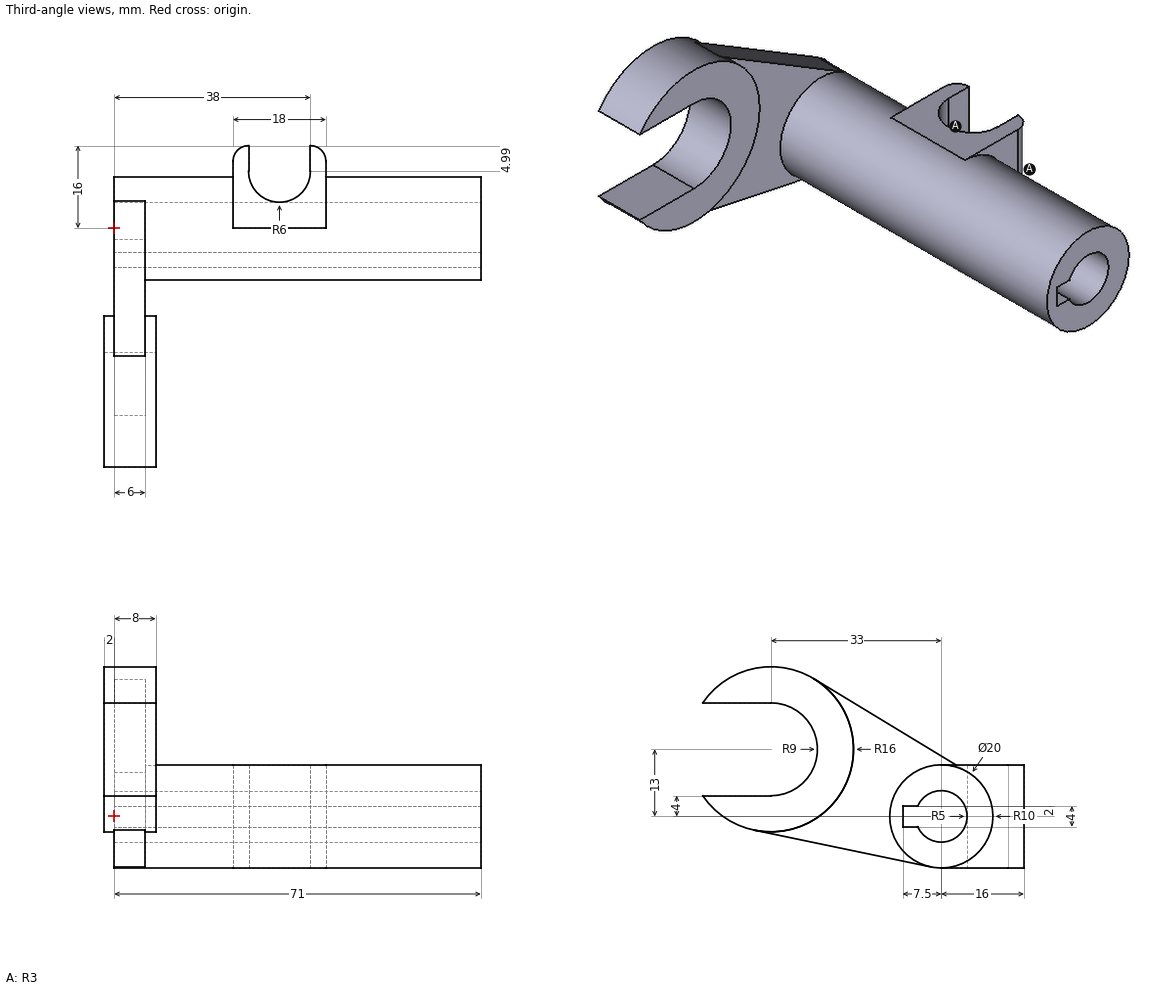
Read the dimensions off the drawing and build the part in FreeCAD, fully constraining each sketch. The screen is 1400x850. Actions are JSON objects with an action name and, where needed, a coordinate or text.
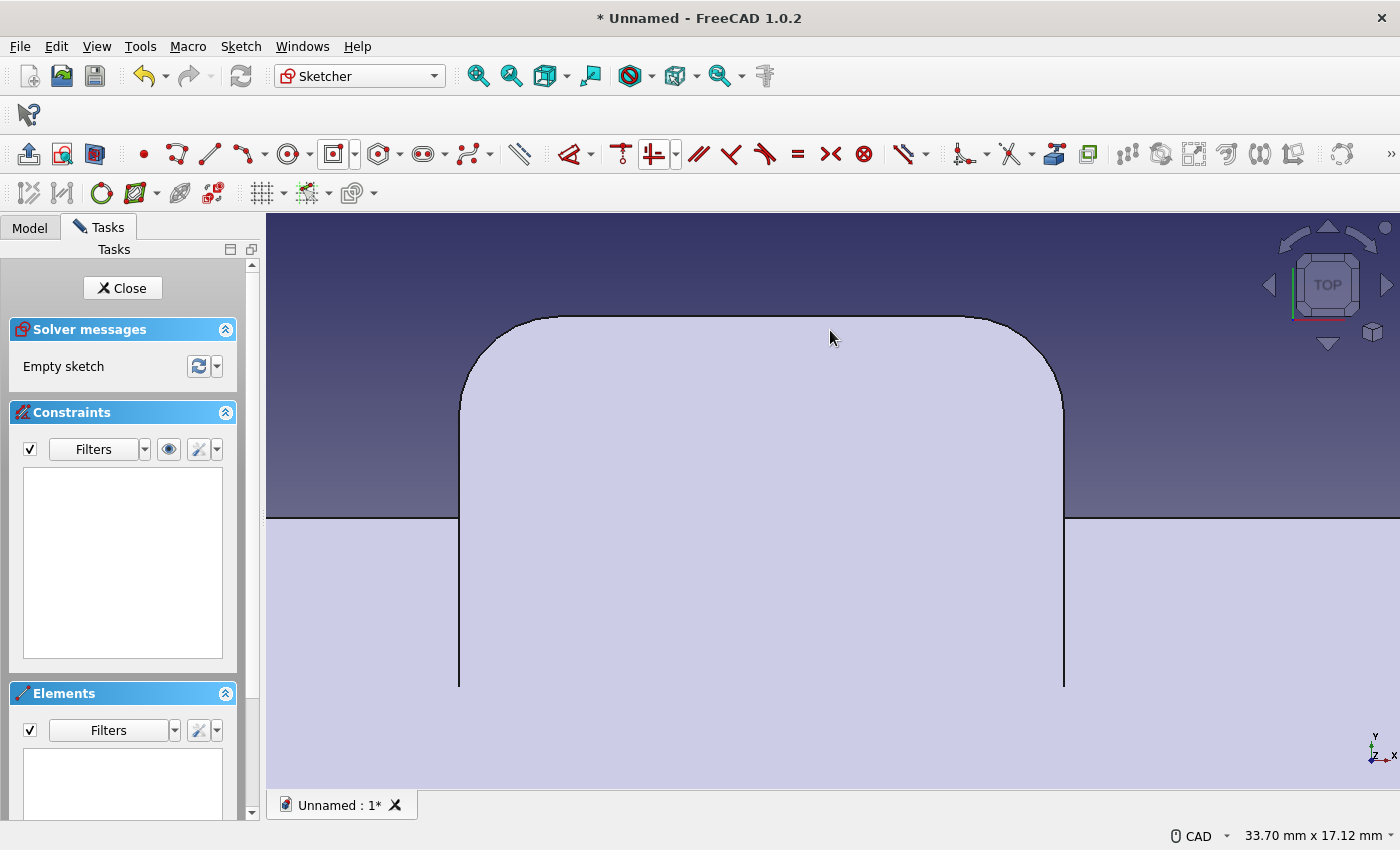
{"action": "left_click", "coordinate": [177, 154]}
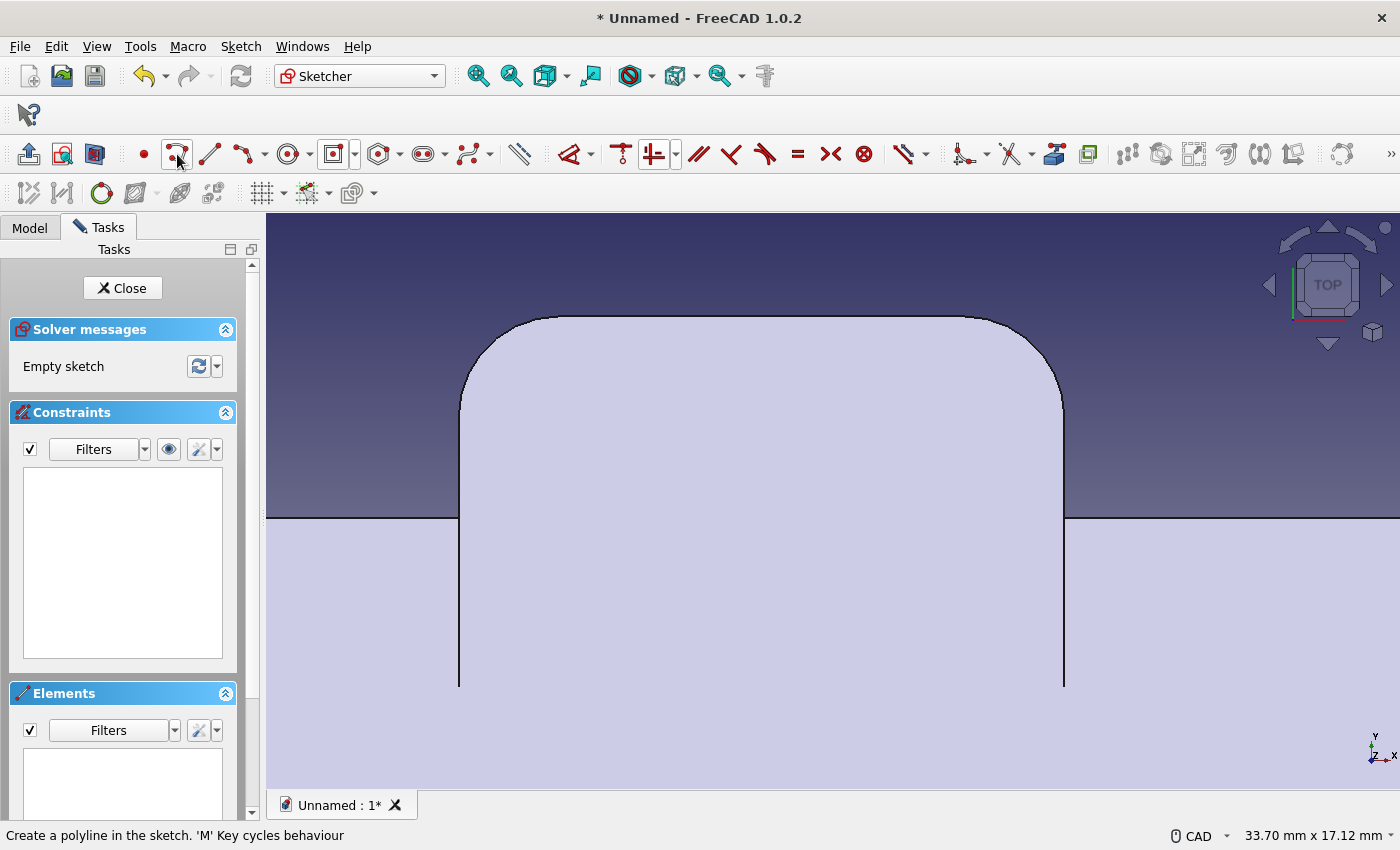
{"action": "left_click", "coordinate": [963, 484]}
{"action": "left_click", "coordinate": [963, 316]}
{"action": "left_click", "coordinate": [560, 316]}
{"action": "left_click", "coordinate": [560, 484]}
{"action": "right_click", "coordinate": [560, 484]}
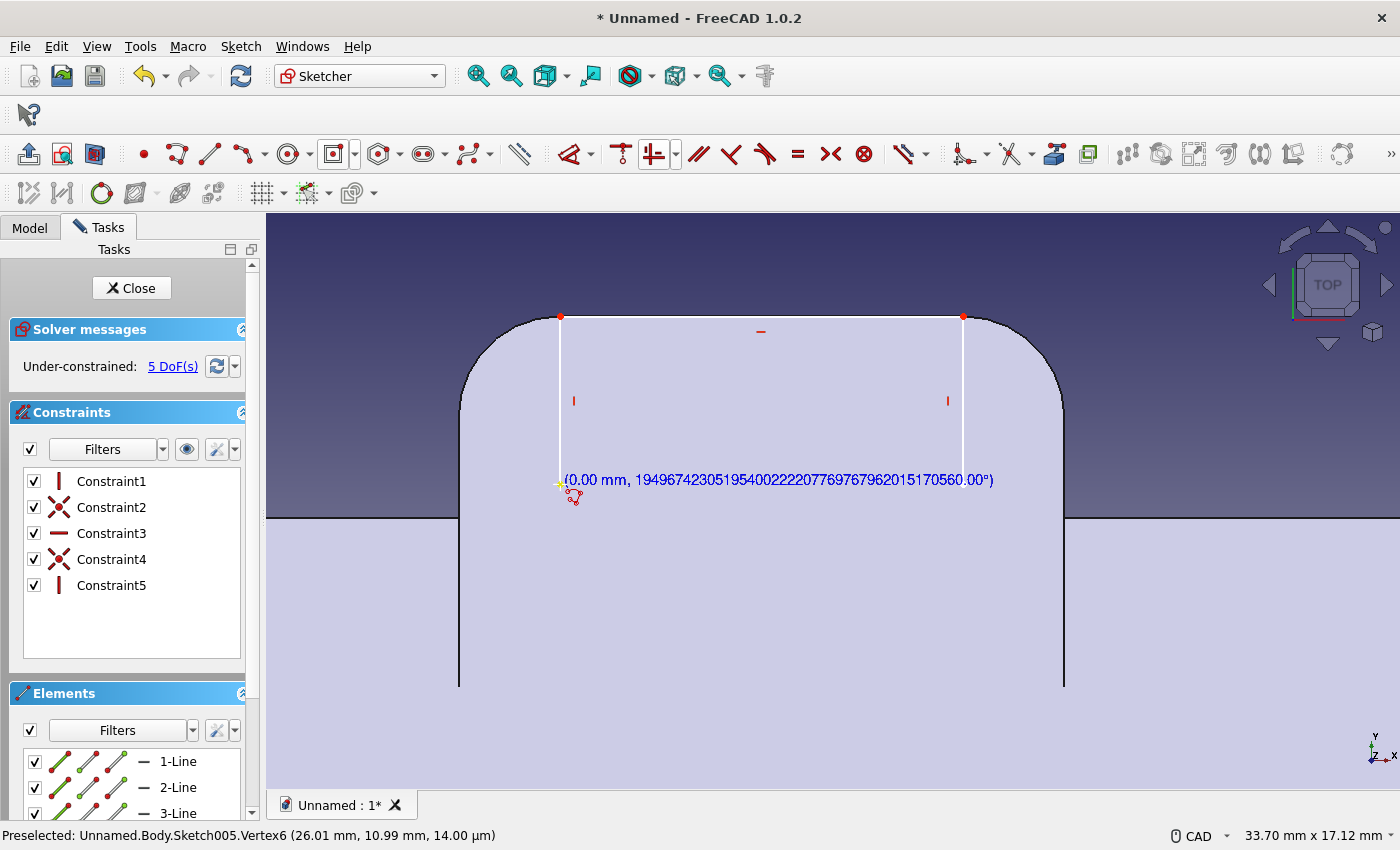
{"action": "key", "text": "g 3 a"}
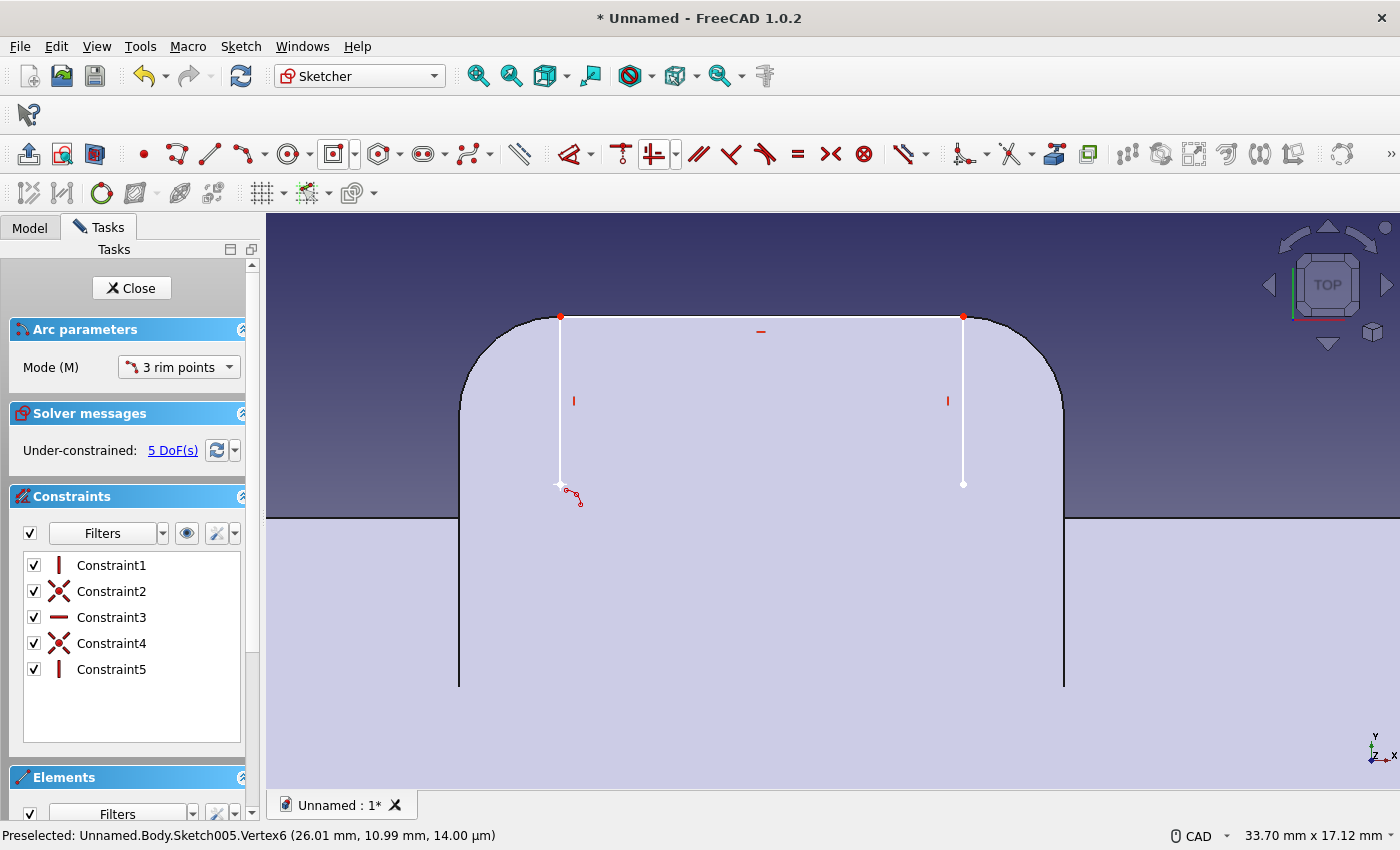
{"action": "left_click", "coordinate": [560, 485]}
{"action": "left_click", "coordinate": [963, 485]}
{"action": "left_click", "coordinate": [762, 686]}
{"action": "key", "text": "Escape"}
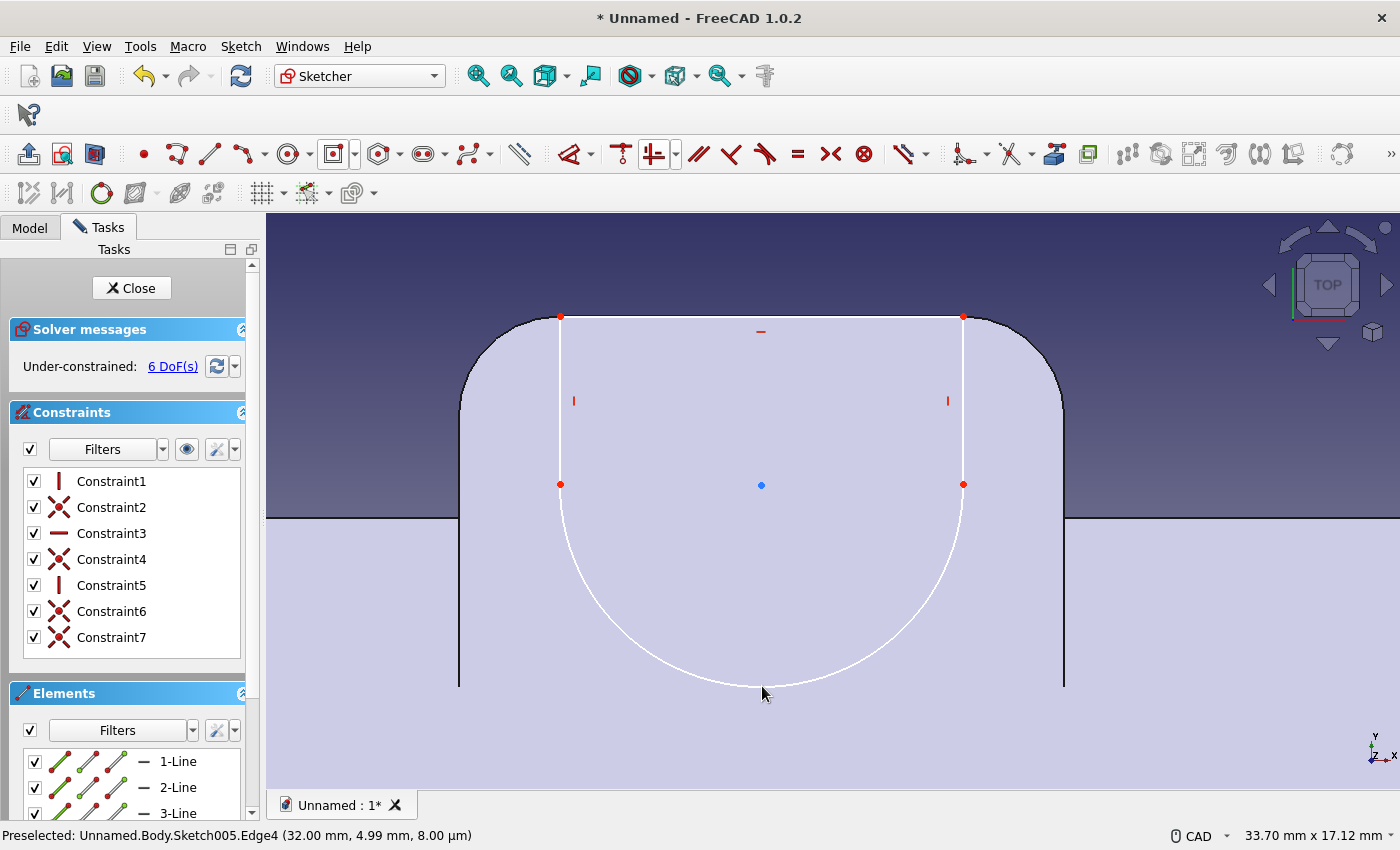
{"action": "left_click", "coordinate": [963, 435]}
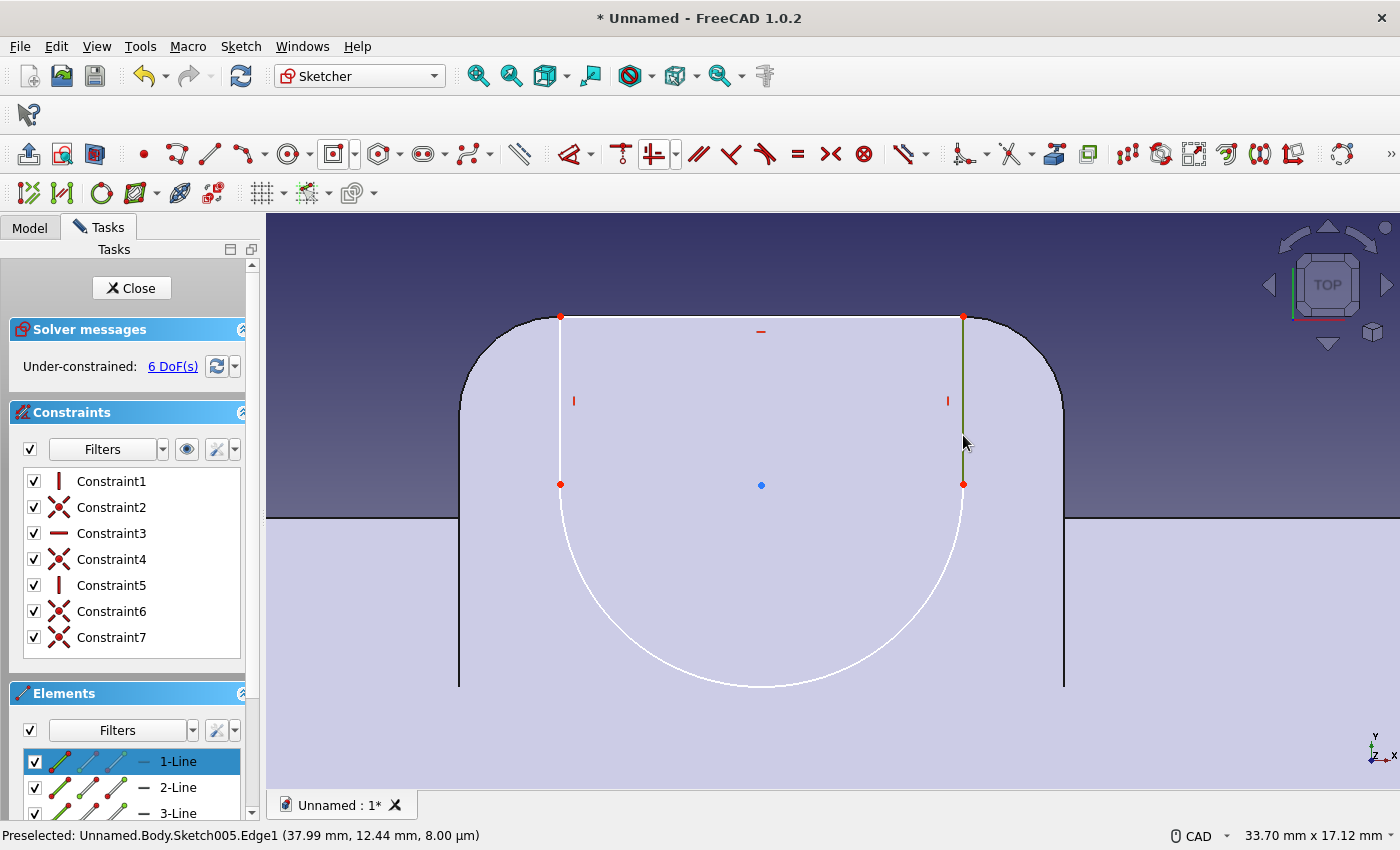
{"action": "left_click", "coordinate": [643, 648]}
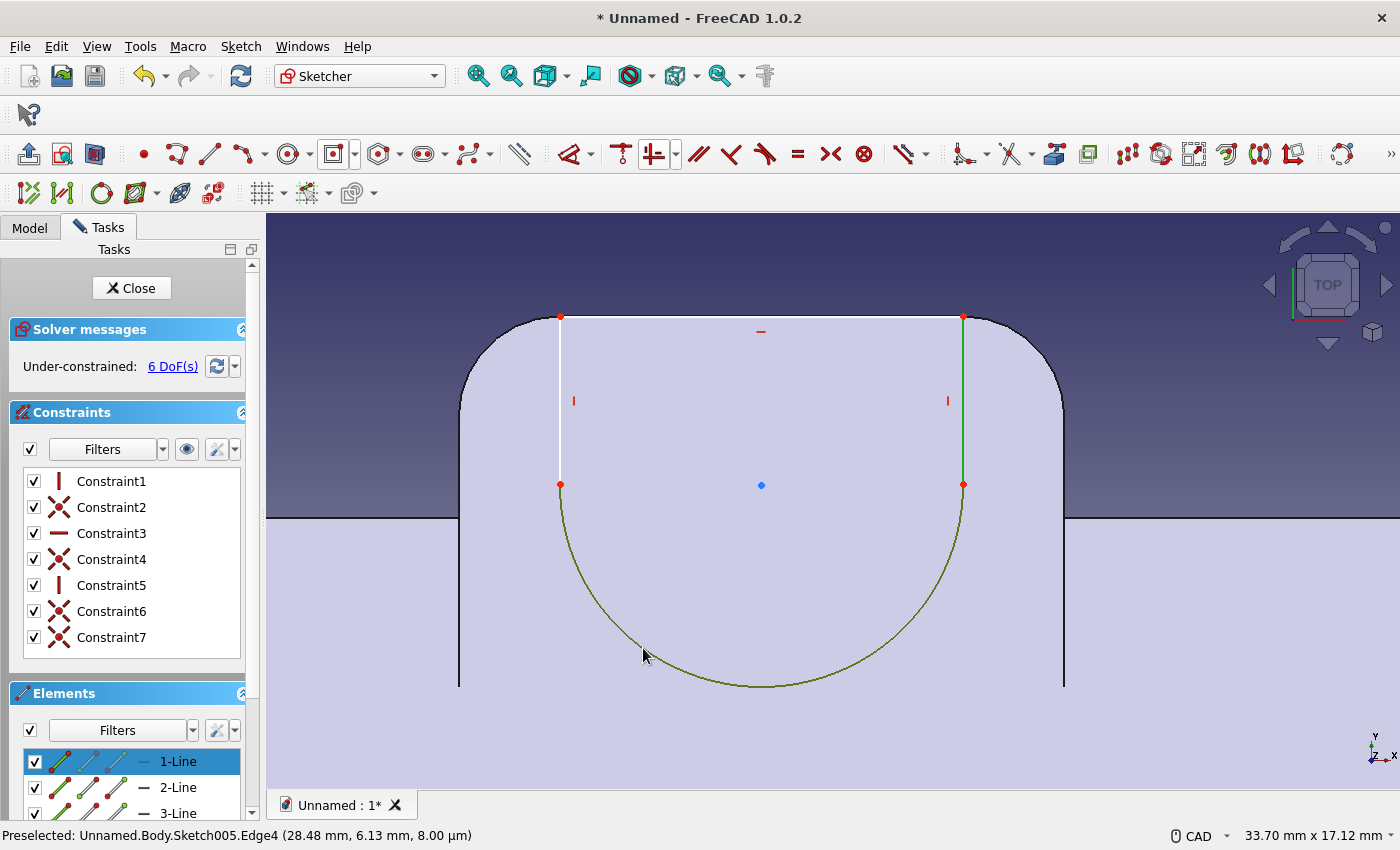
{"action": "key", "text": "t"}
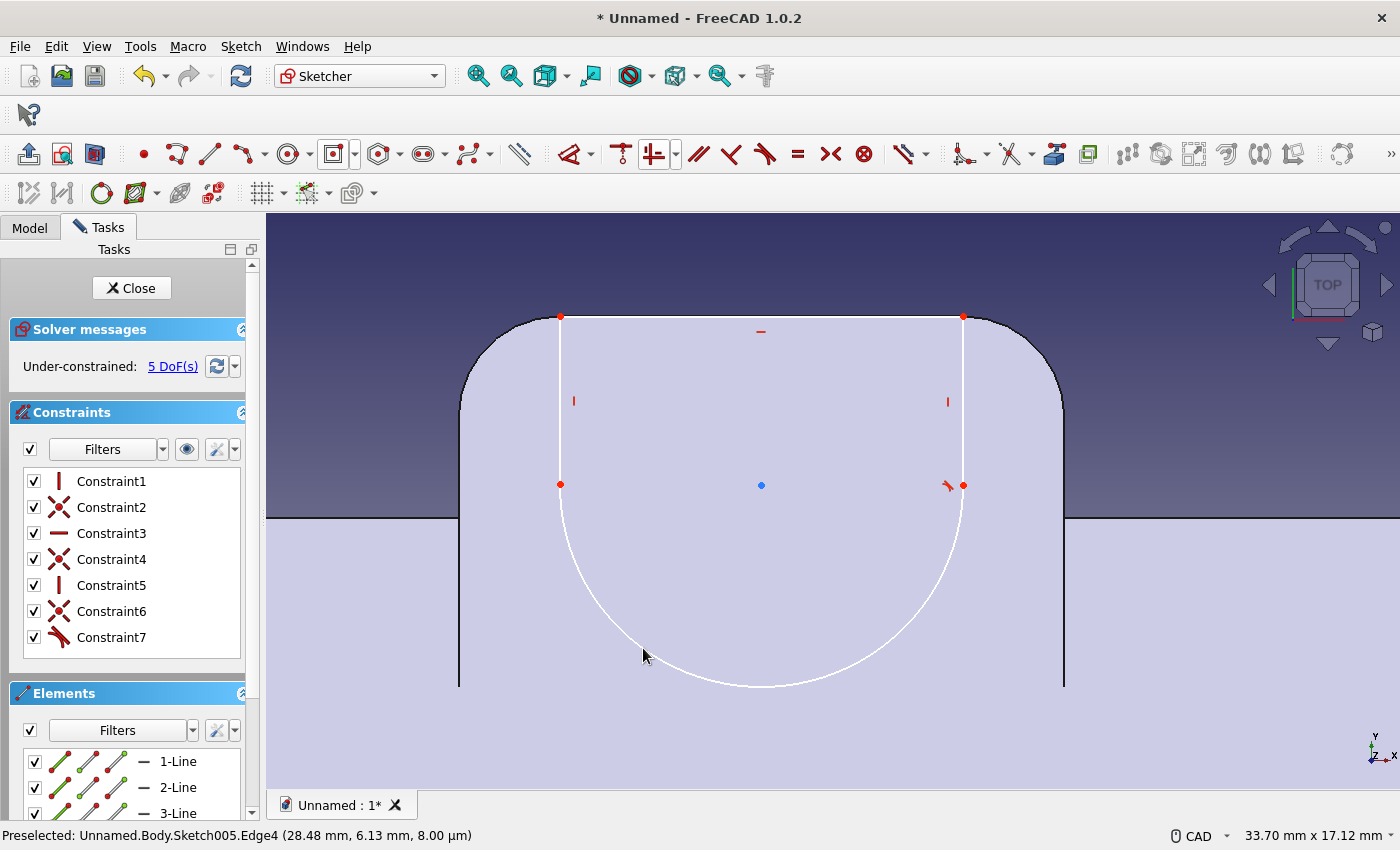
{"action": "left_click", "coordinate": [560, 367]}